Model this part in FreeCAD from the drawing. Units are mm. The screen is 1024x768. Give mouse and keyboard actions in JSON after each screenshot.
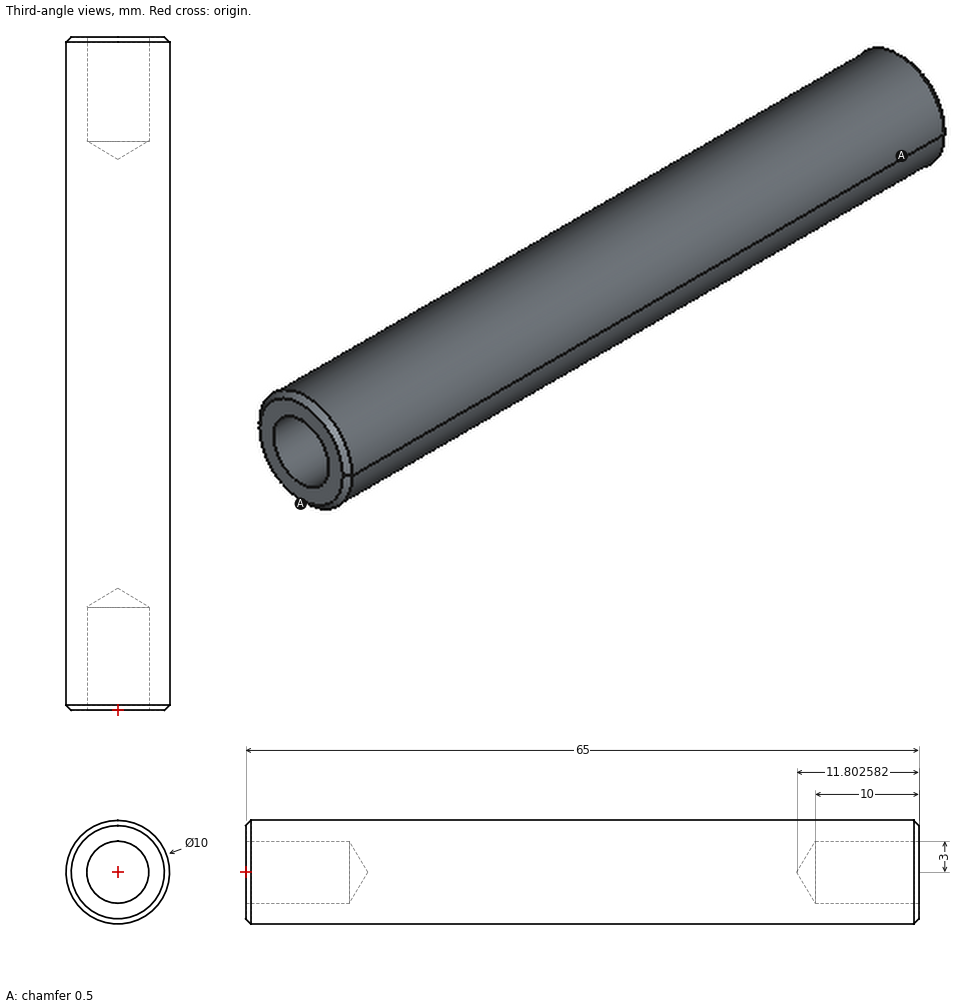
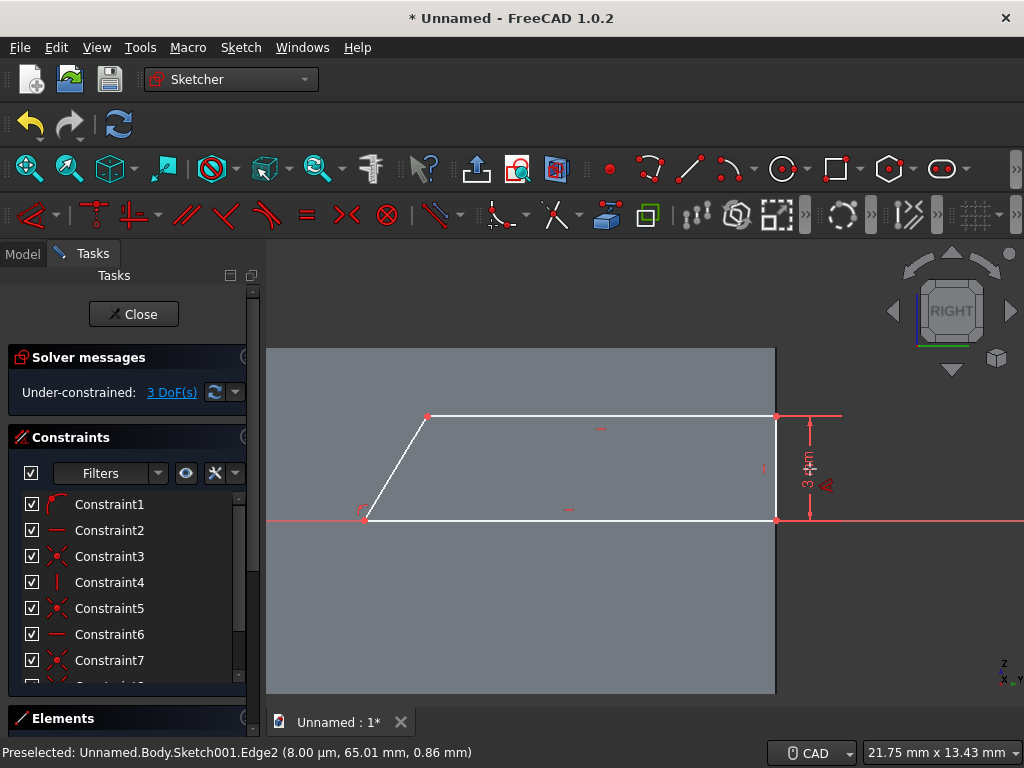
{"action": "left_click", "coordinate": [671, 416]}
{"action": "left_click", "coordinate": [601, 382]}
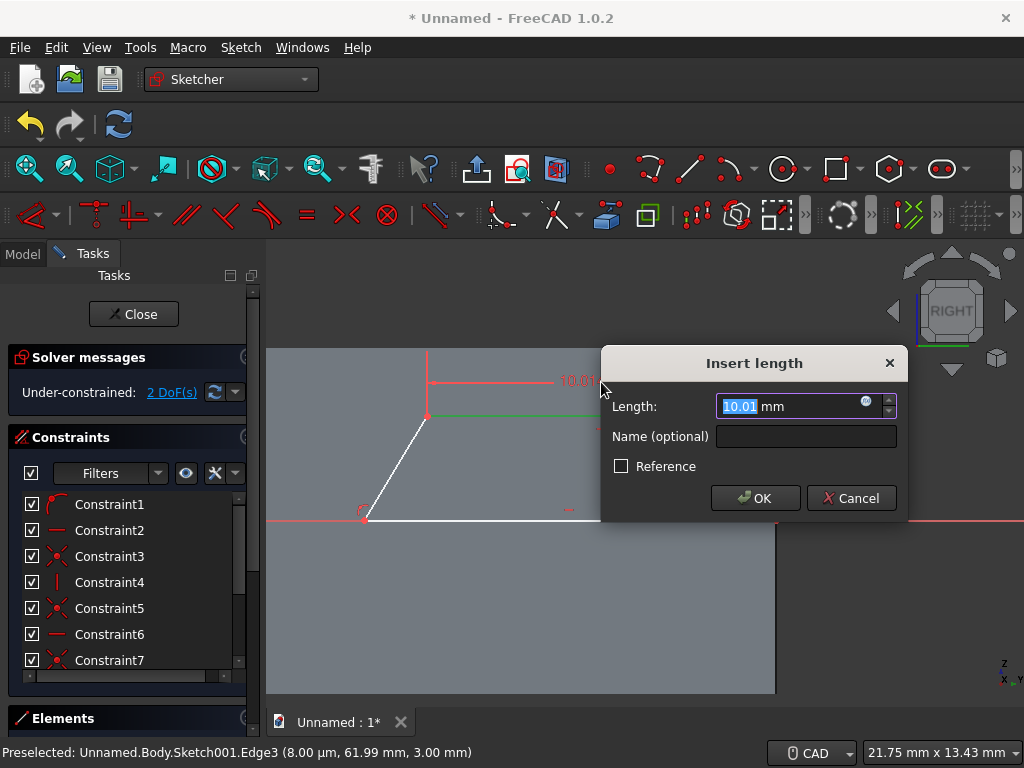
{"action": "type", "text": "10"}
{"action": "key", "text": "Return"}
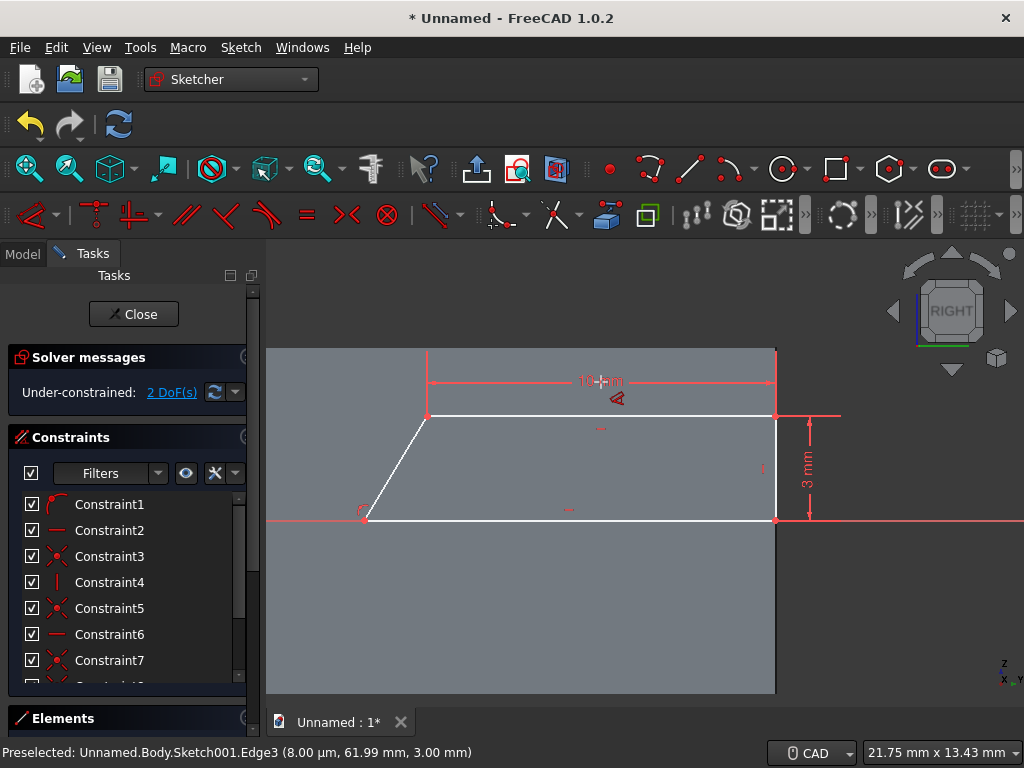
{"action": "left_click", "coordinate": [776, 521]}
{"action": "left_click", "coordinate": [535, 555]}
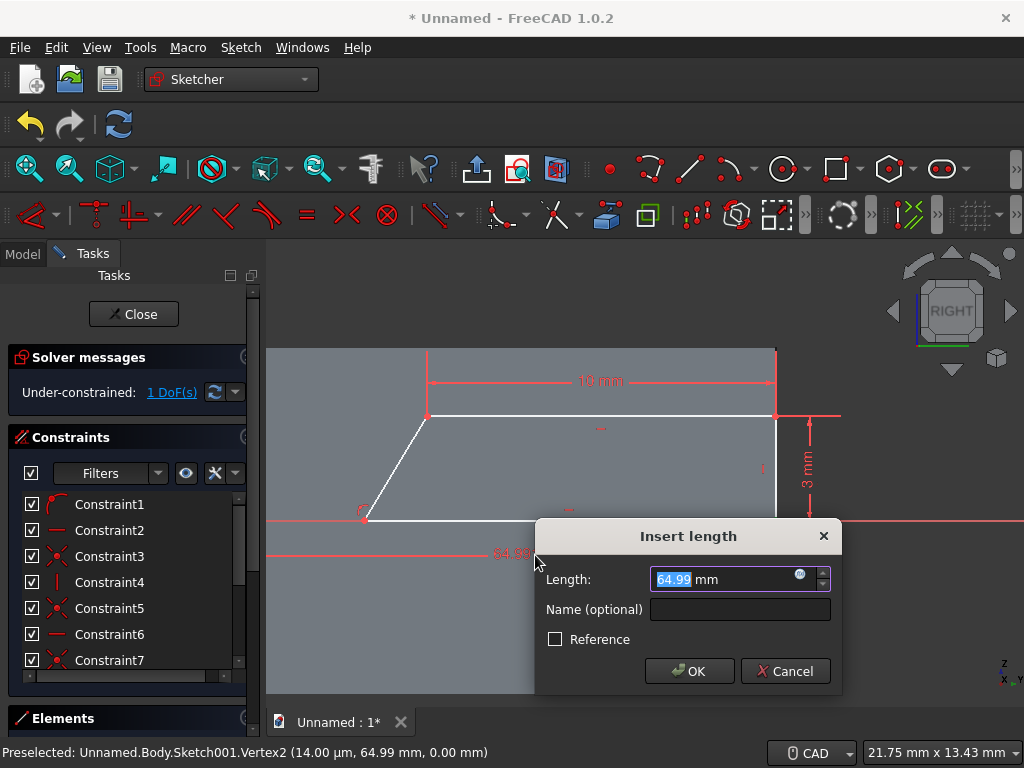
{"action": "type", "text": "65"}
{"action": "key", "text": "Return"}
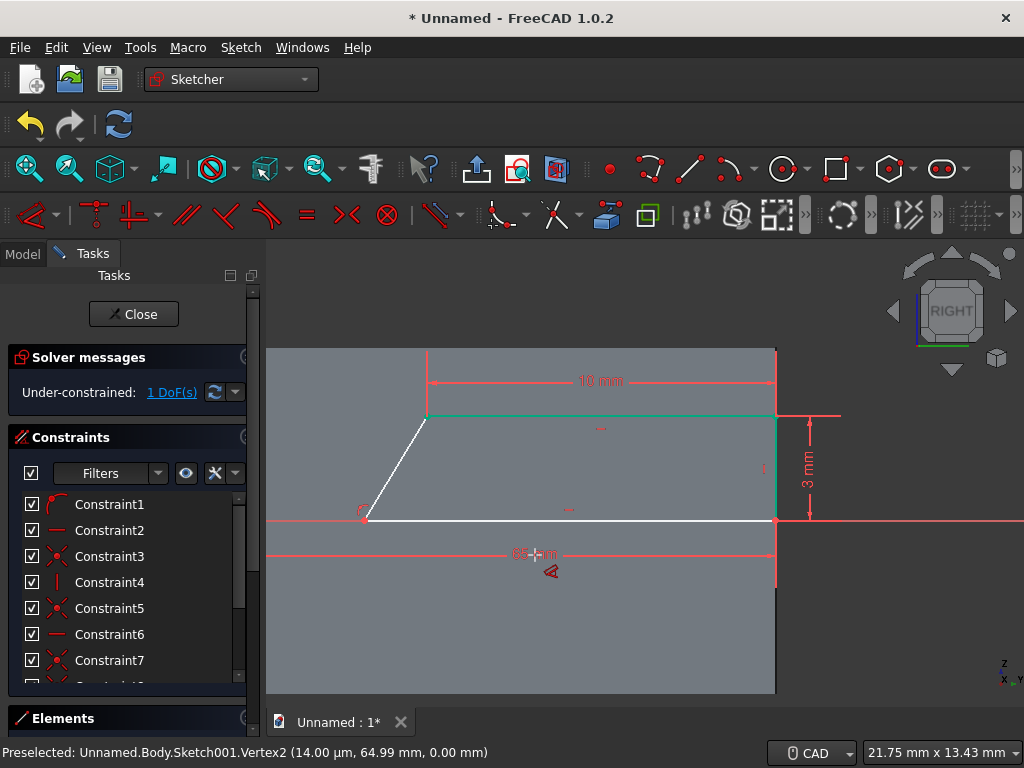
{"action": "left_click", "coordinate": [488, 521]}
{"action": "left_click", "coordinate": [665, 555]}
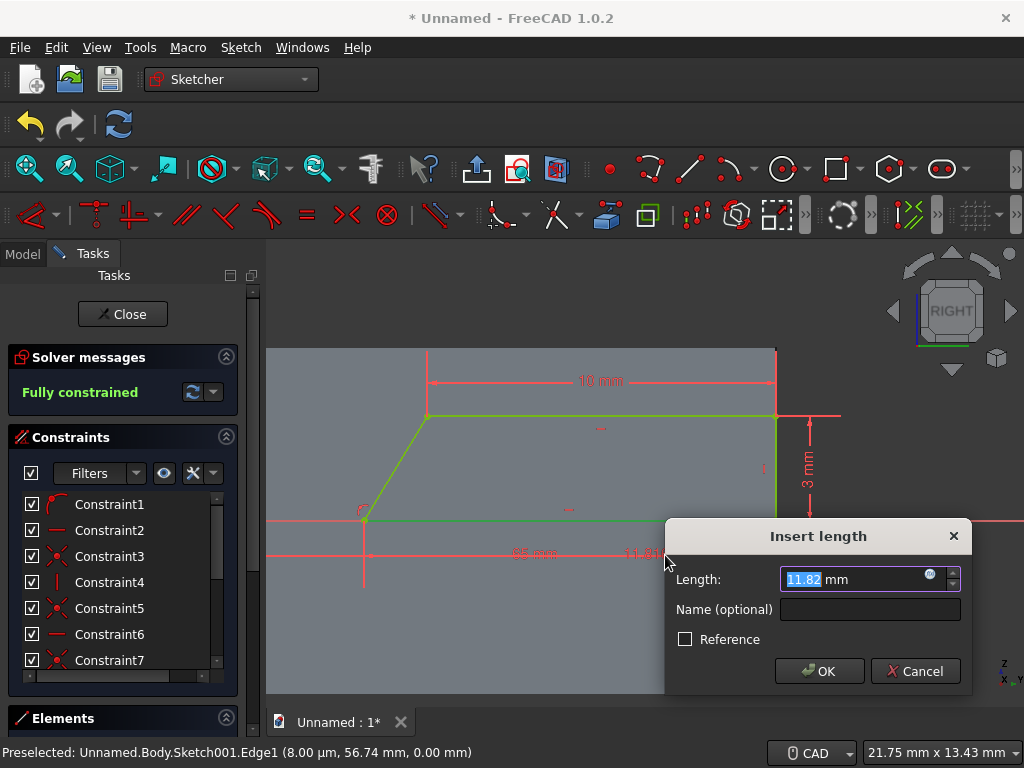
{"action": "type", "text": "11.802582"}
{"action": "key", "text": "Return"}
{"action": "key", "text": "Escape"}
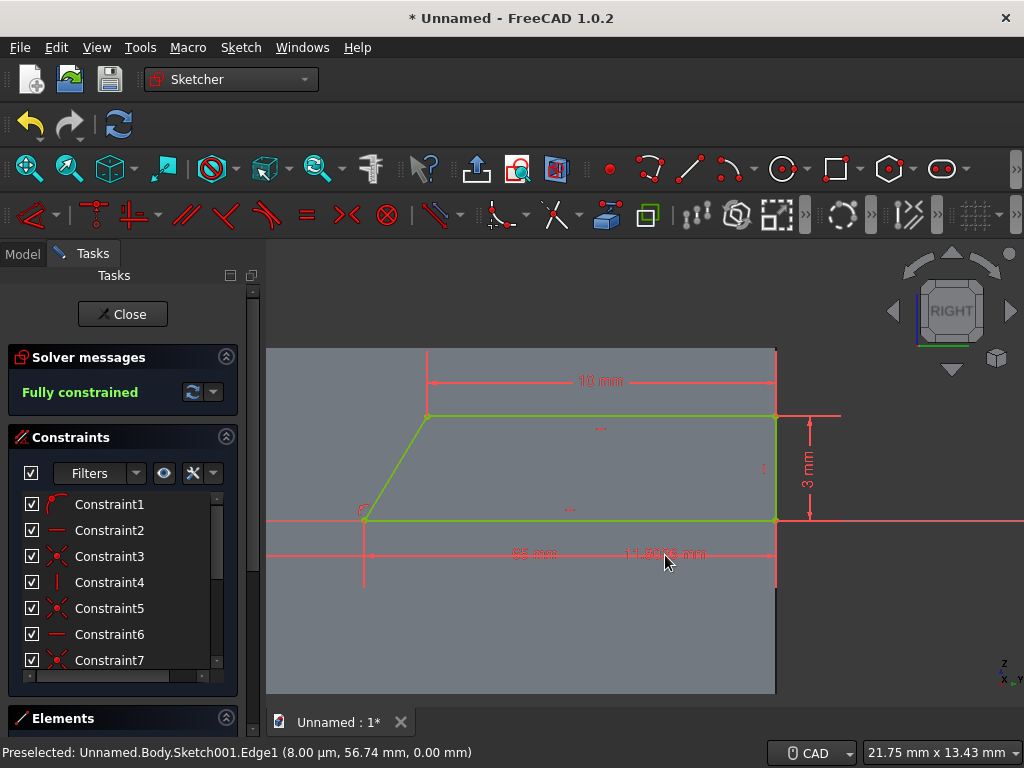
{"action": "left_click", "coordinate": [123, 314]}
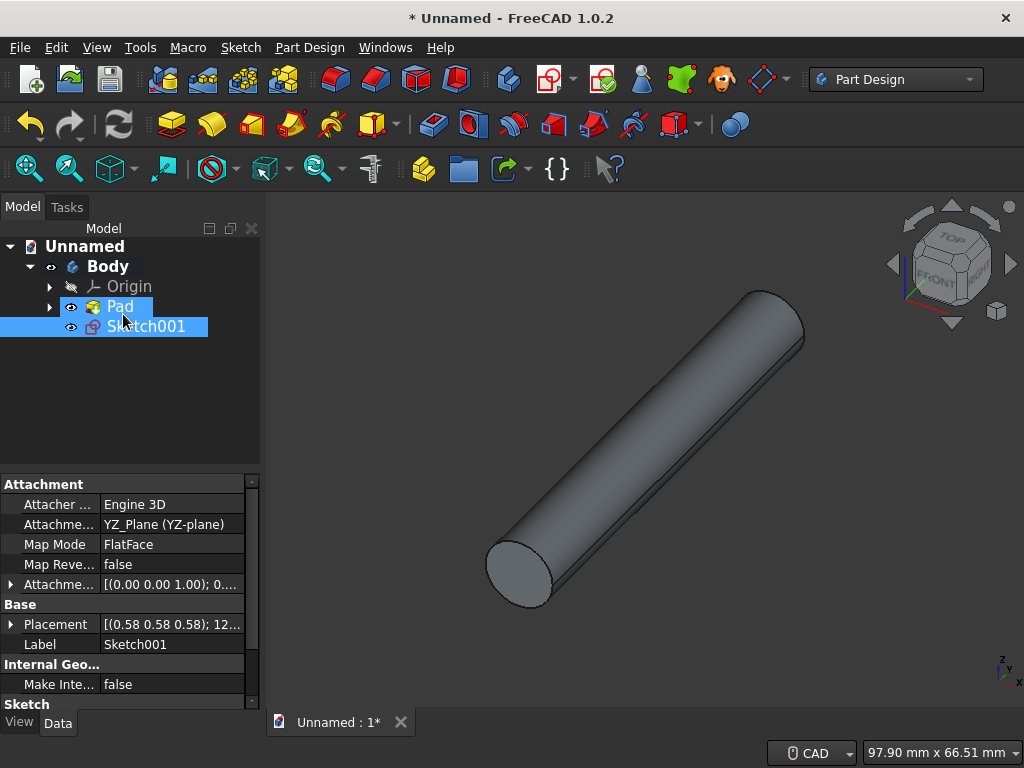
{"action": "left_click", "coordinate": [514, 124]}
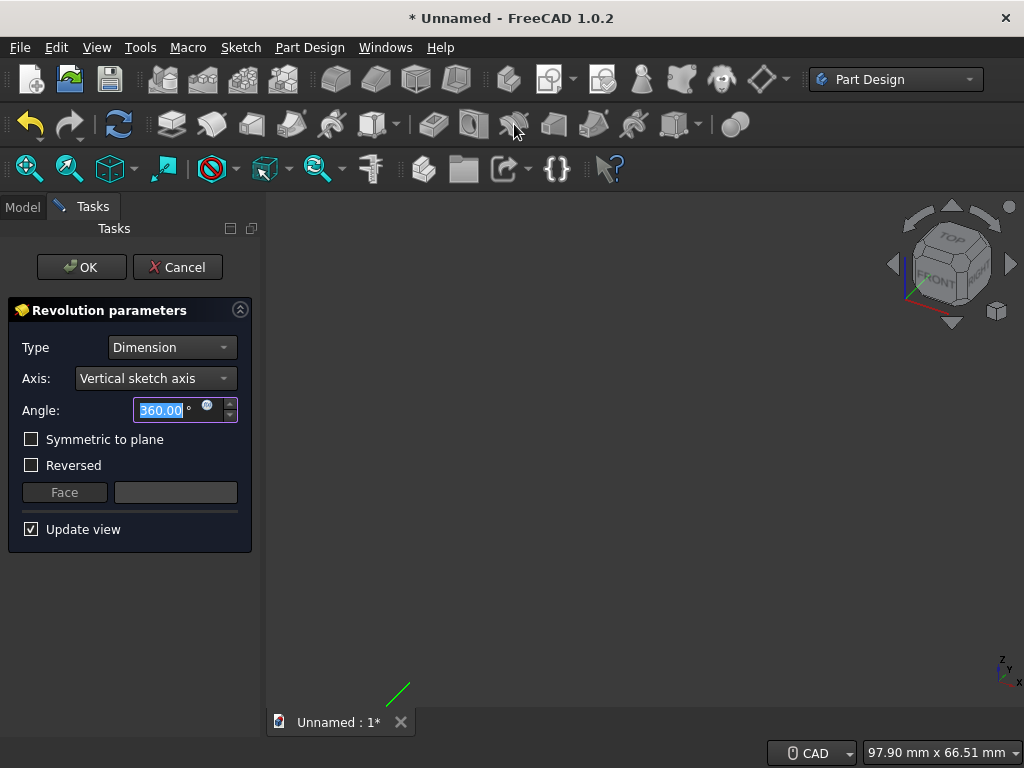
{"action": "left_click", "coordinate": [156, 378]}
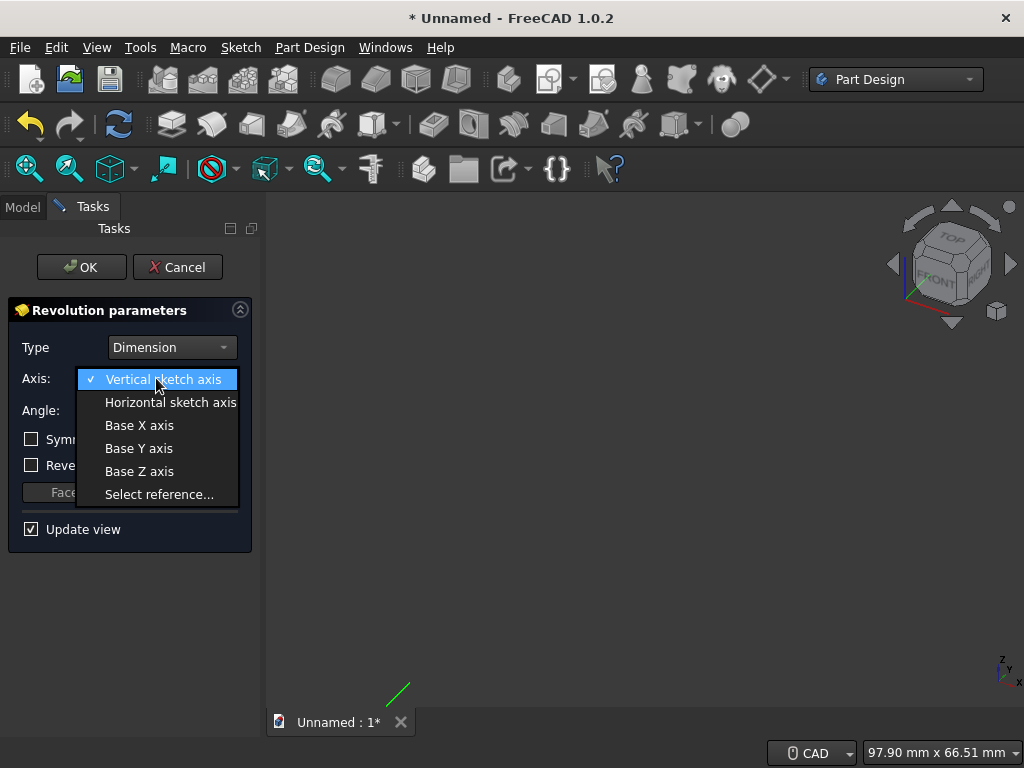
{"action": "left_click", "coordinate": [156, 402]}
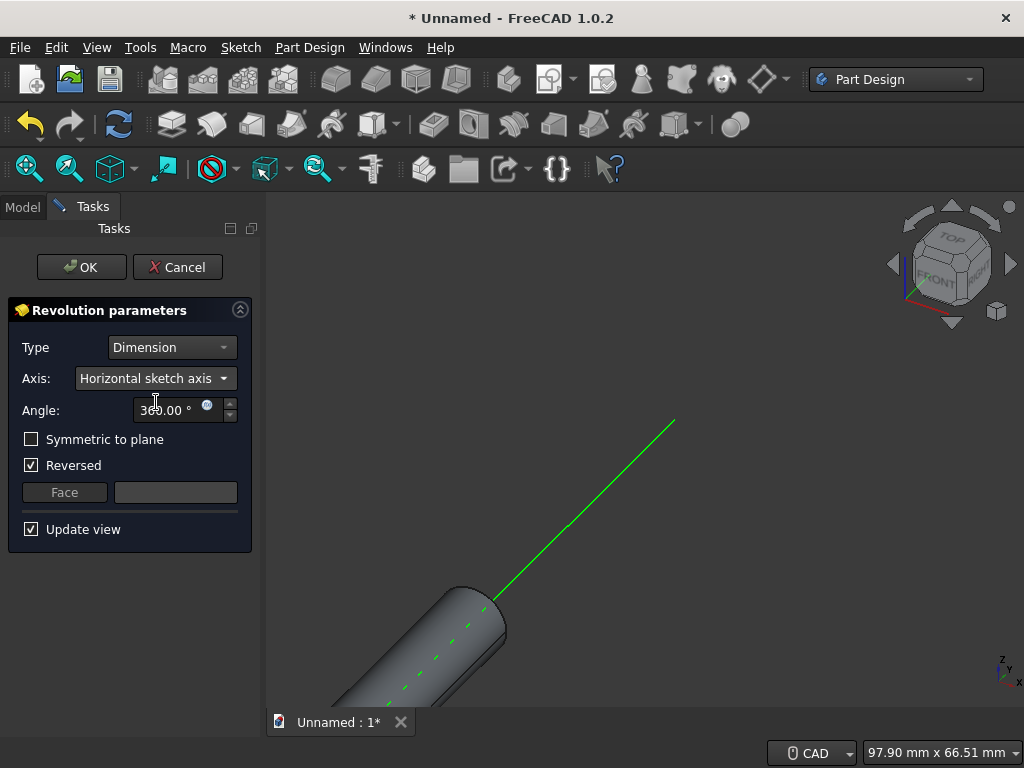
{"action": "left_click", "coordinate": [82, 267]}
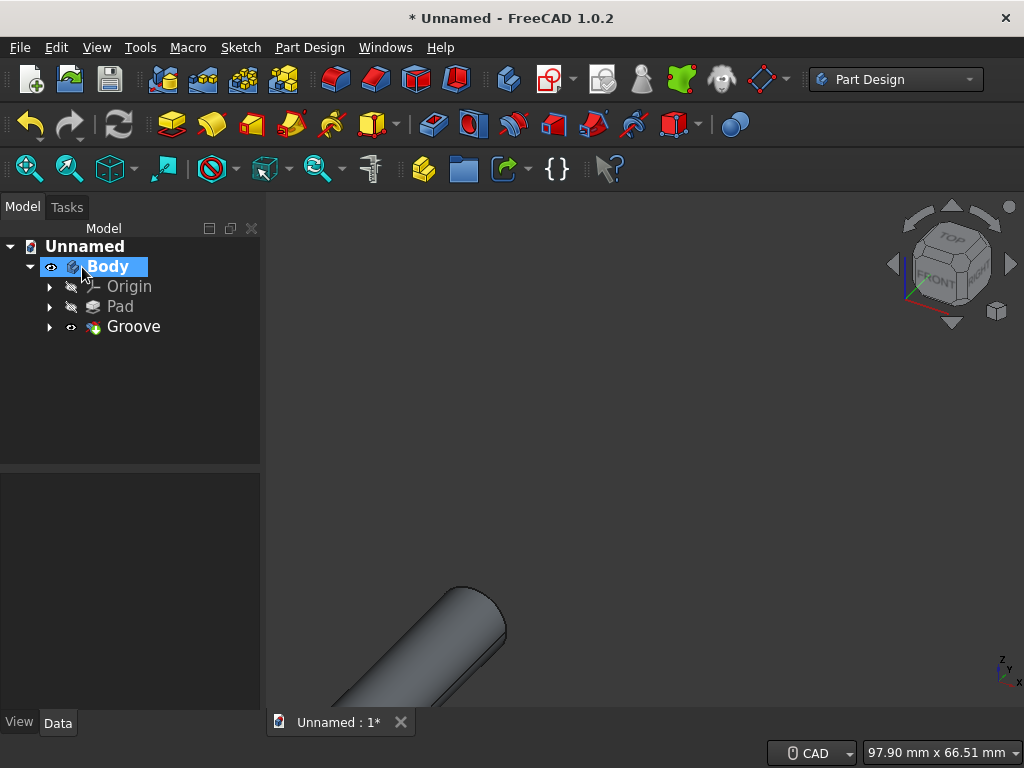
{"action": "left_click", "coordinate": [30, 170]}